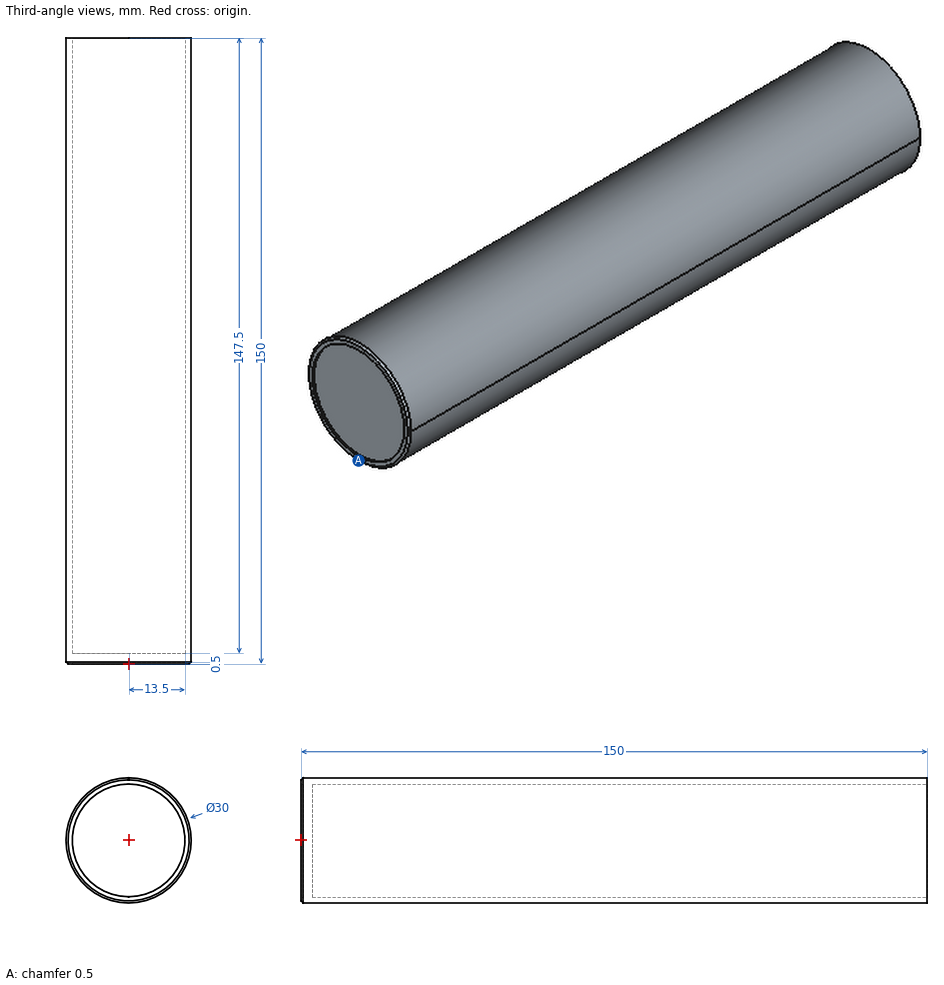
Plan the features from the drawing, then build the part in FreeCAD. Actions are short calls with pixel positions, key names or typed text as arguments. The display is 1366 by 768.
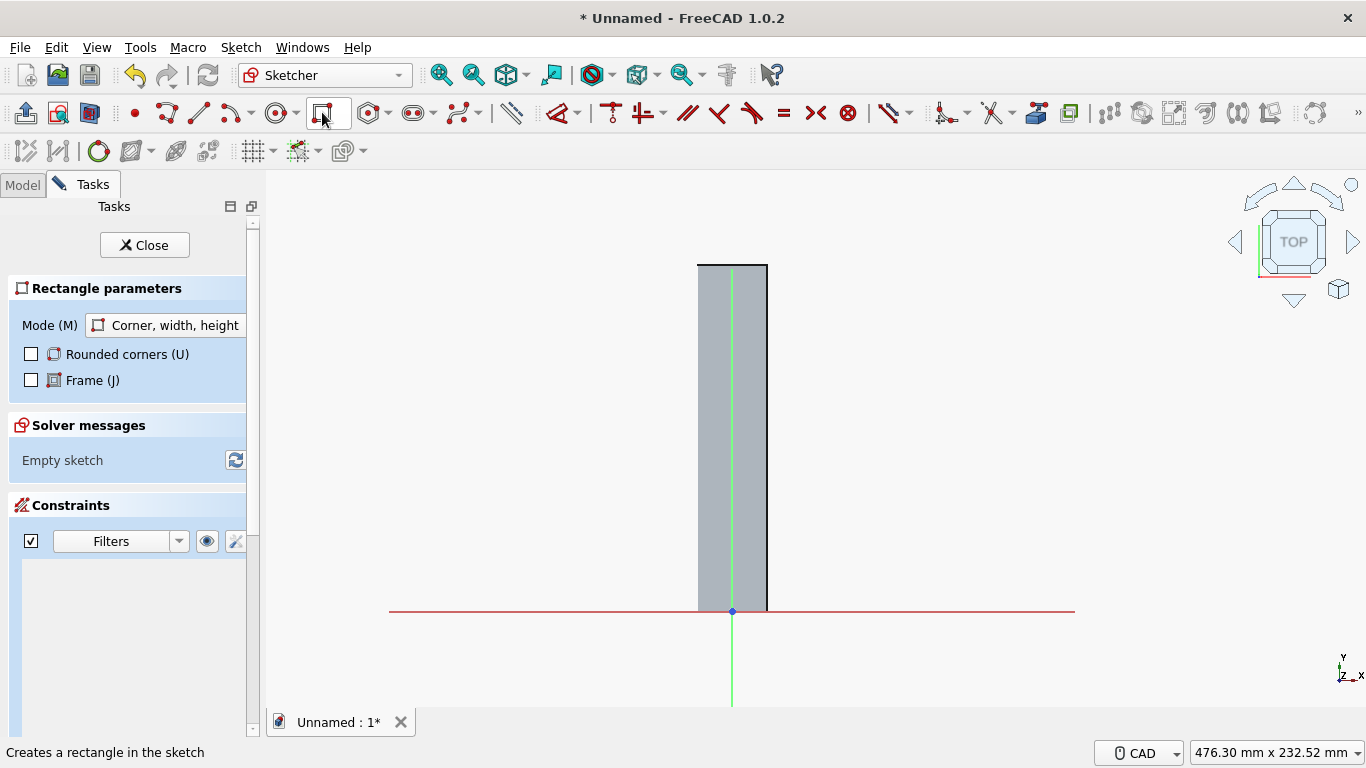
click(732, 265)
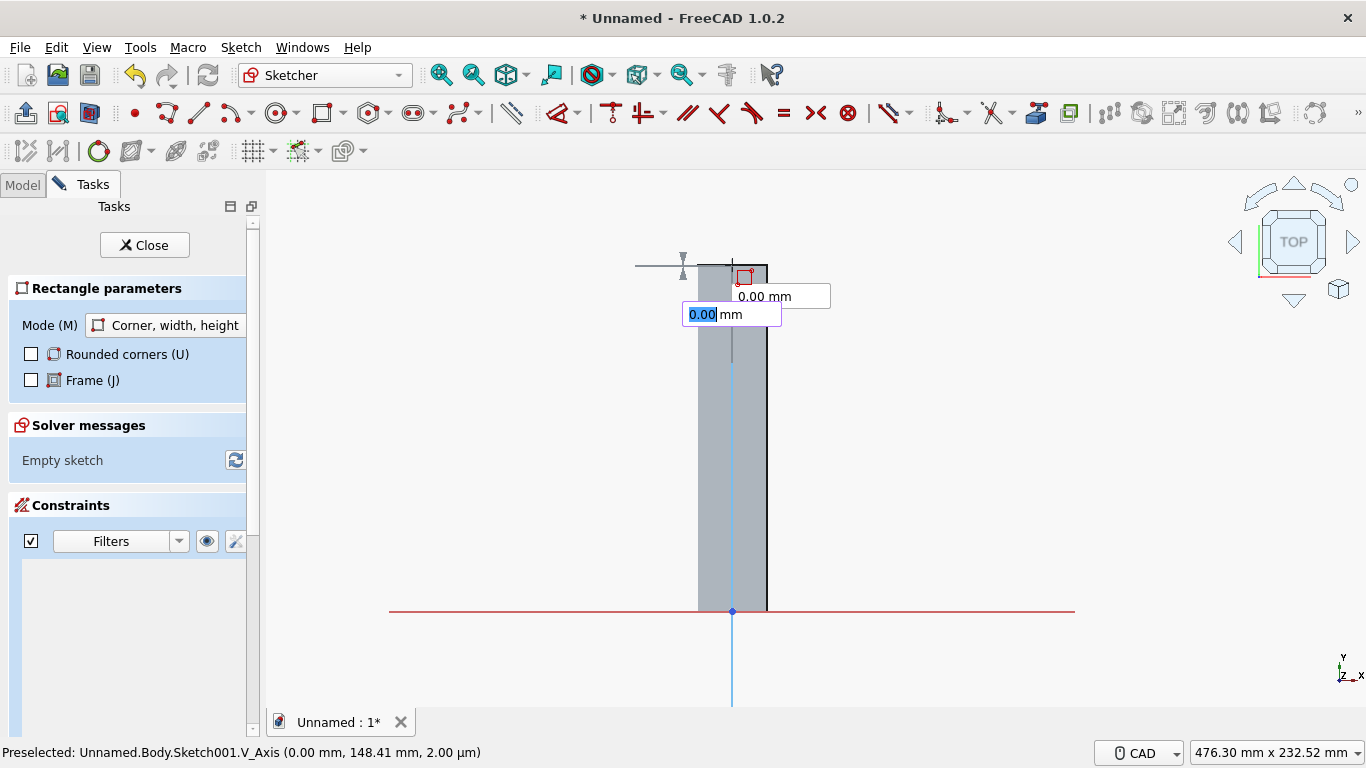
scroll(763, 606, up, 6)
move(763, 604)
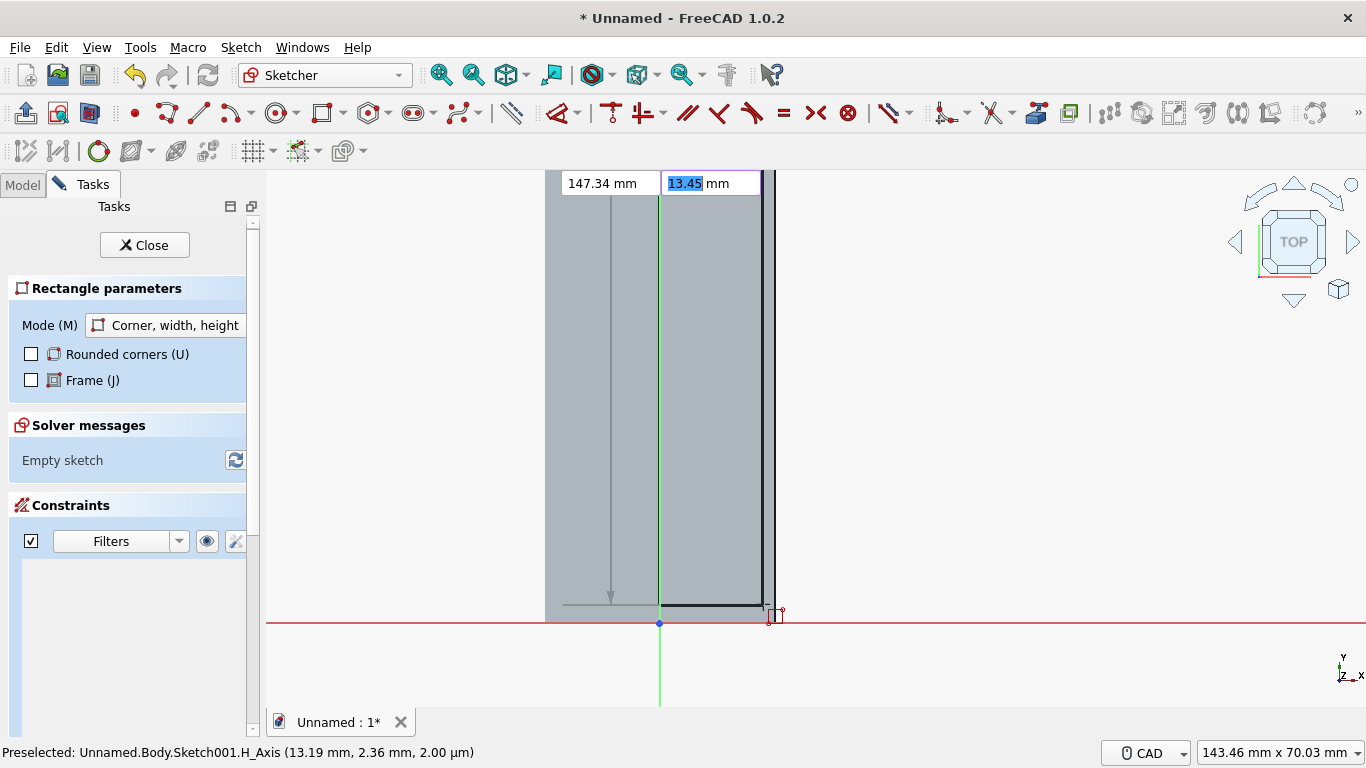
text(13.5)
key(Tab)
text(147.5)
key(Return)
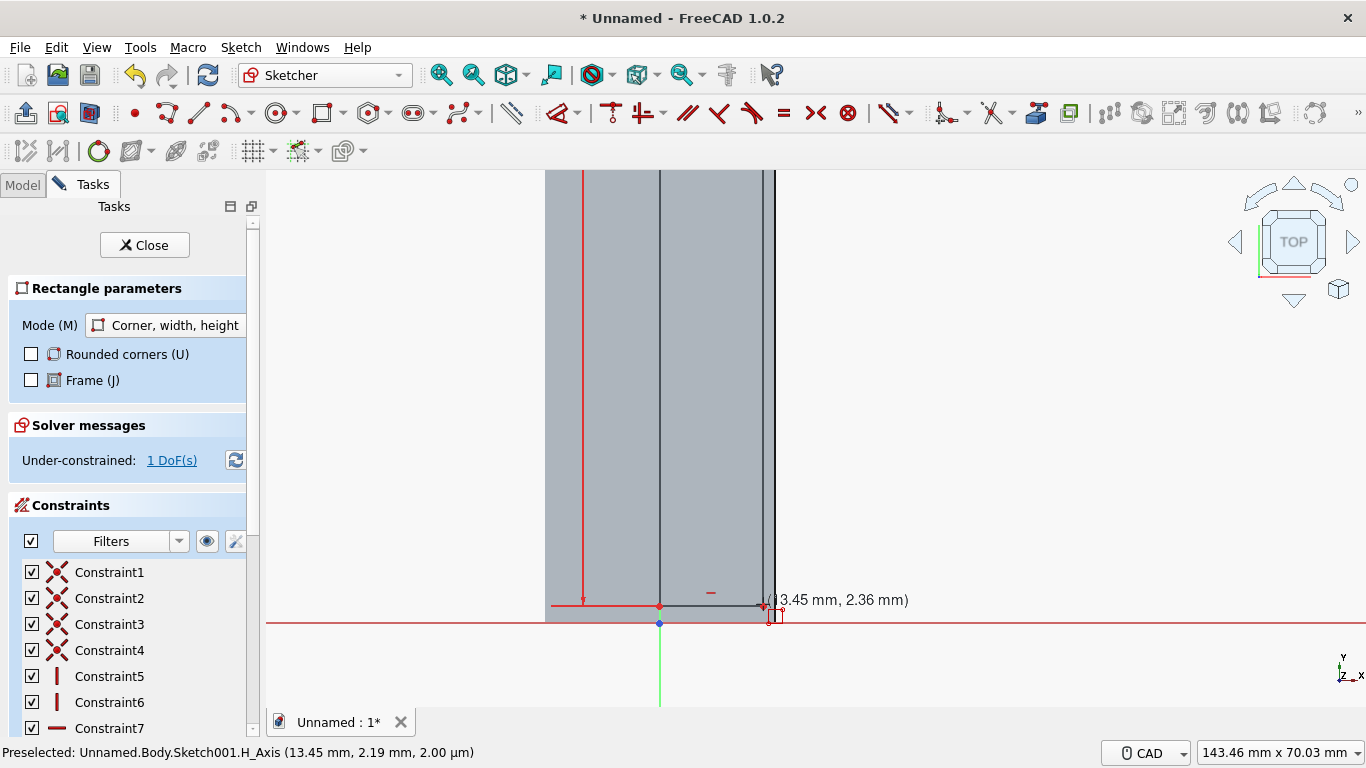
scroll(660, 623, up, 8)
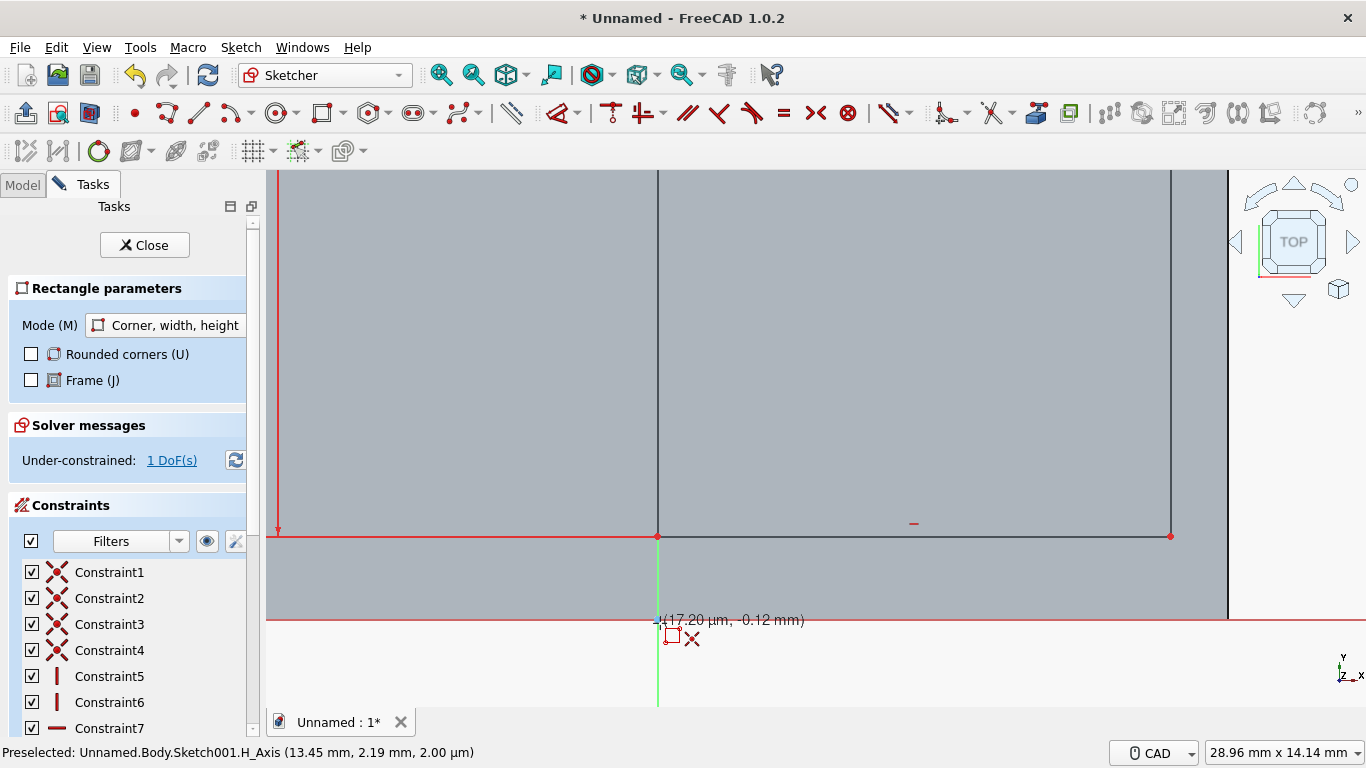
scroll(737, 611, down, 14)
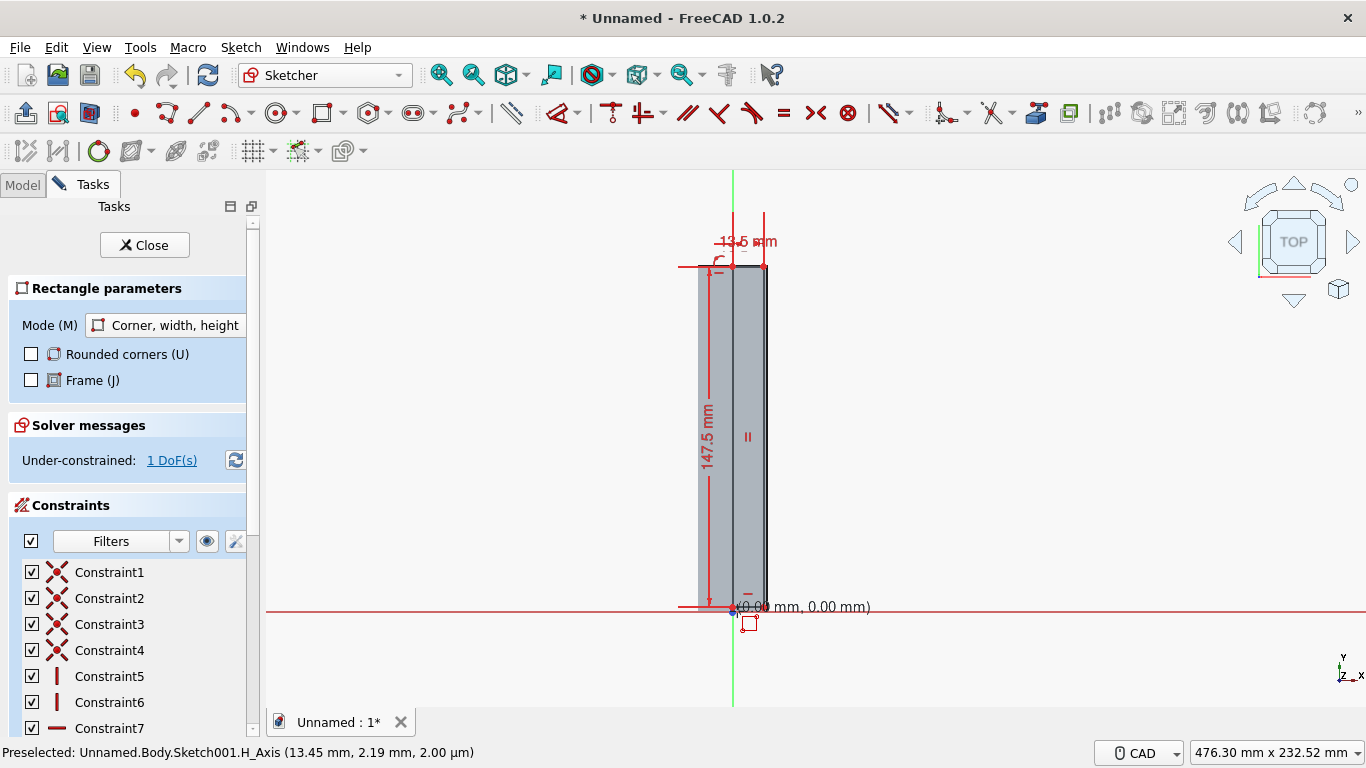
scroll(733, 612, up, 6)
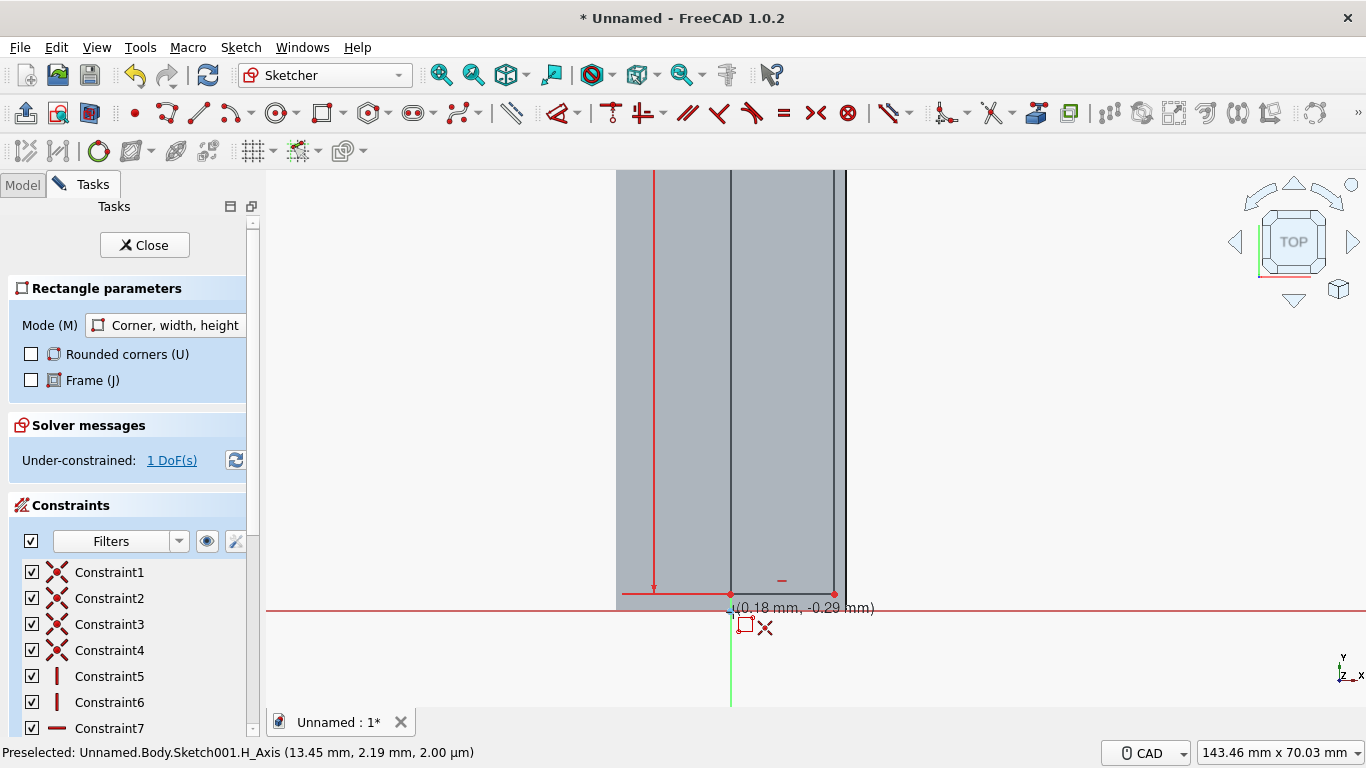
click(731, 611)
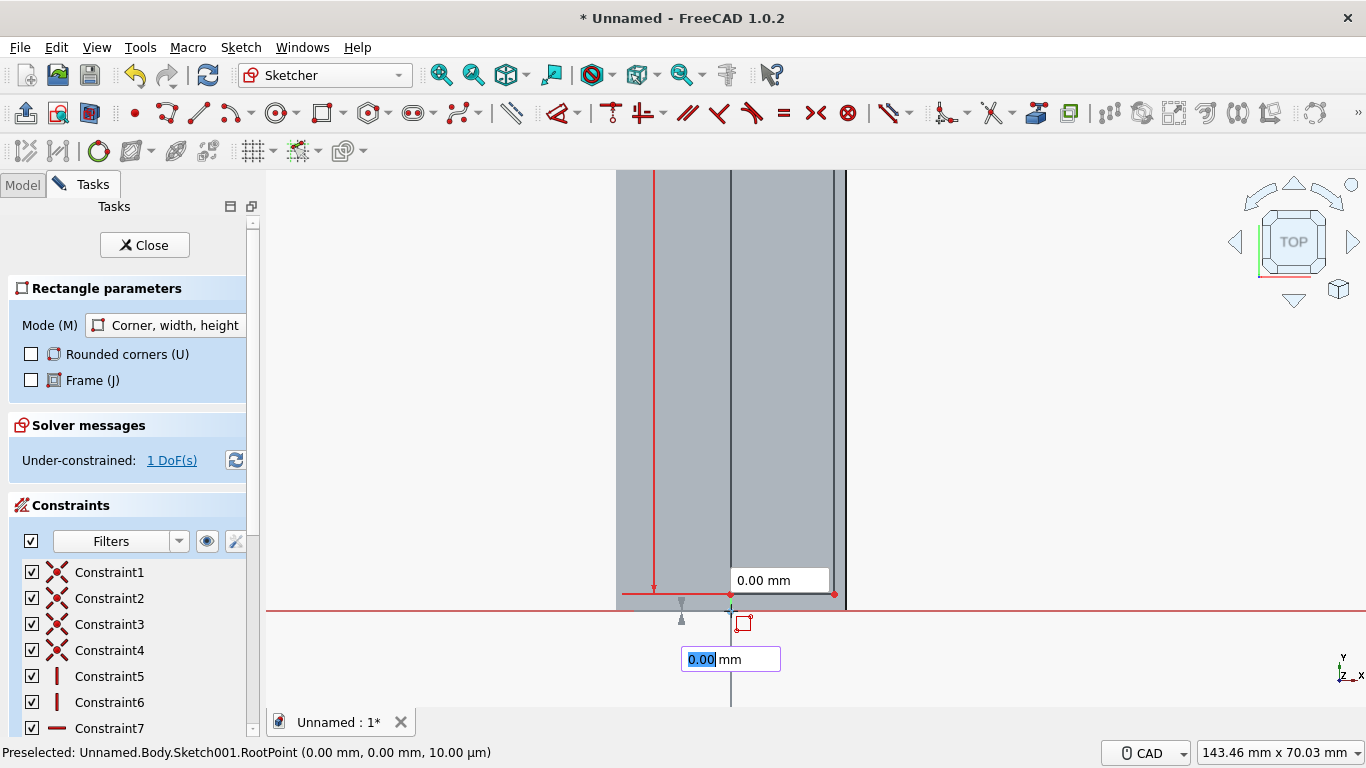
scroll(834, 607, up, 8)
move(833, 605)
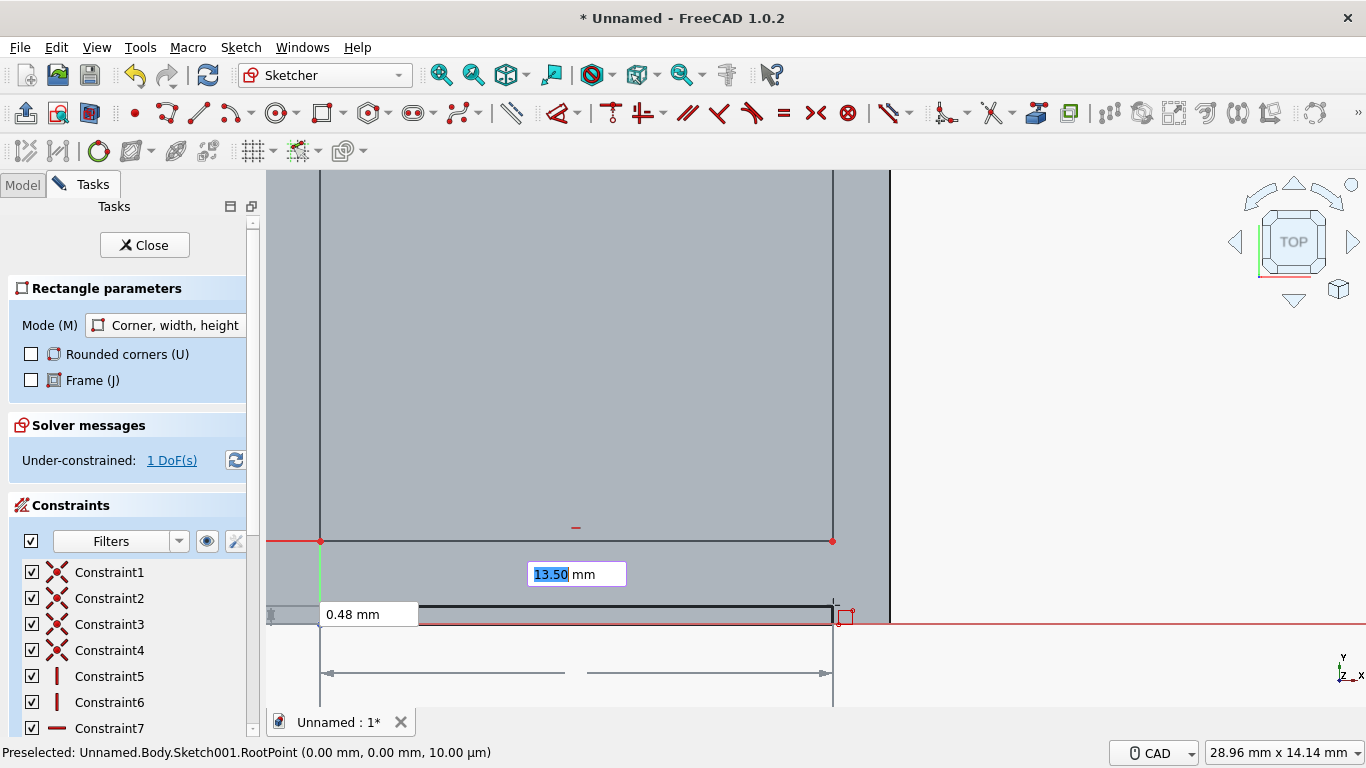
text(13.5)
key(Tab)
text(0.5)
key(Return)
key(Escape)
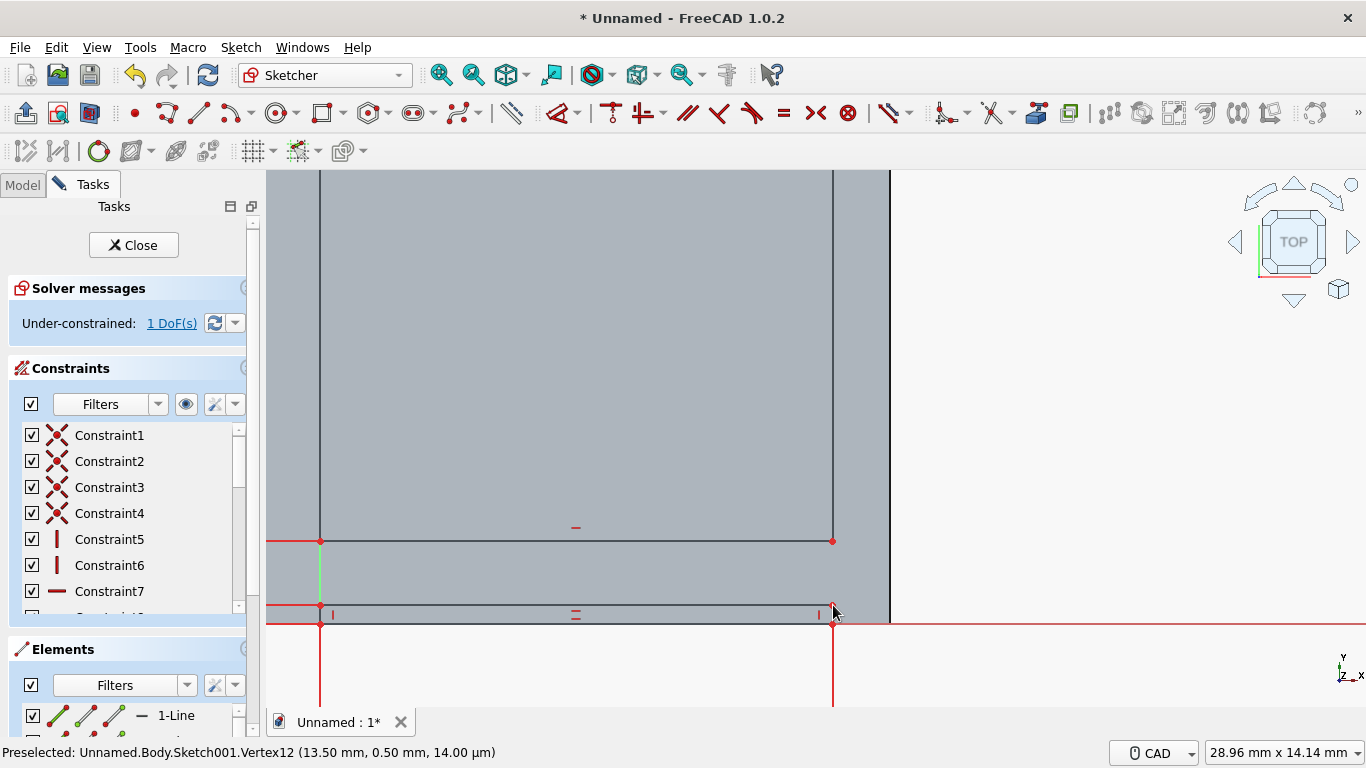
click(558, 114)